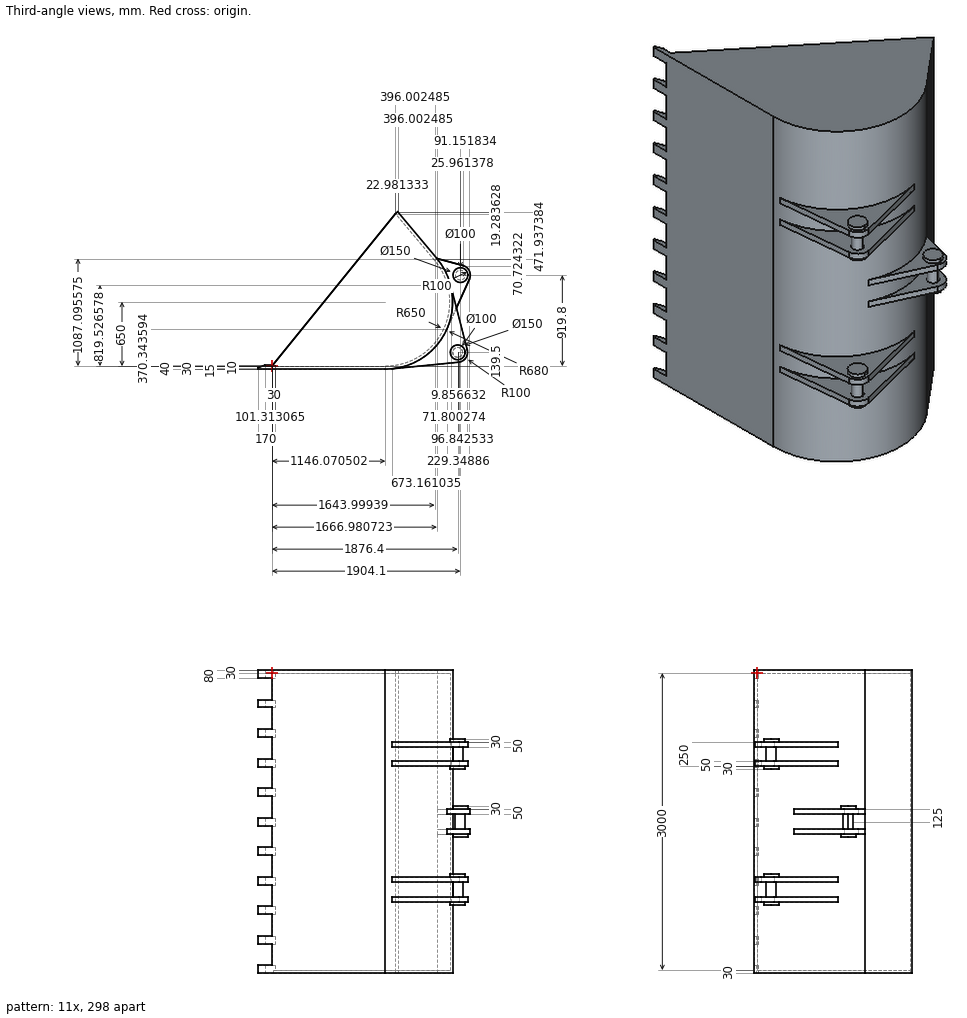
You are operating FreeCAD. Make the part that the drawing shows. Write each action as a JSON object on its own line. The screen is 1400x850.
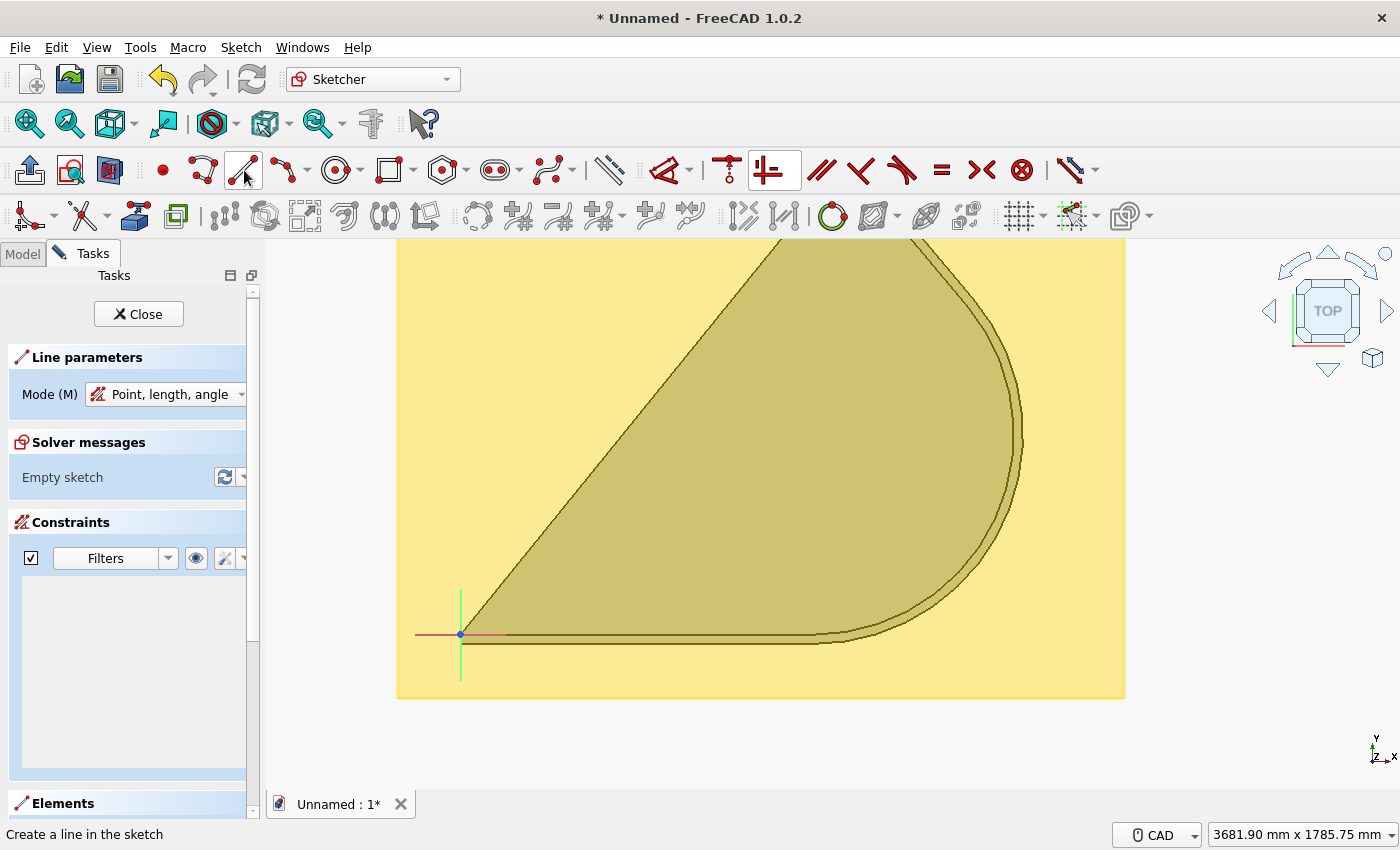
{"action": "scroll", "coordinate": [834, 643], "scroll_direction": "up", "scroll_amount": 4}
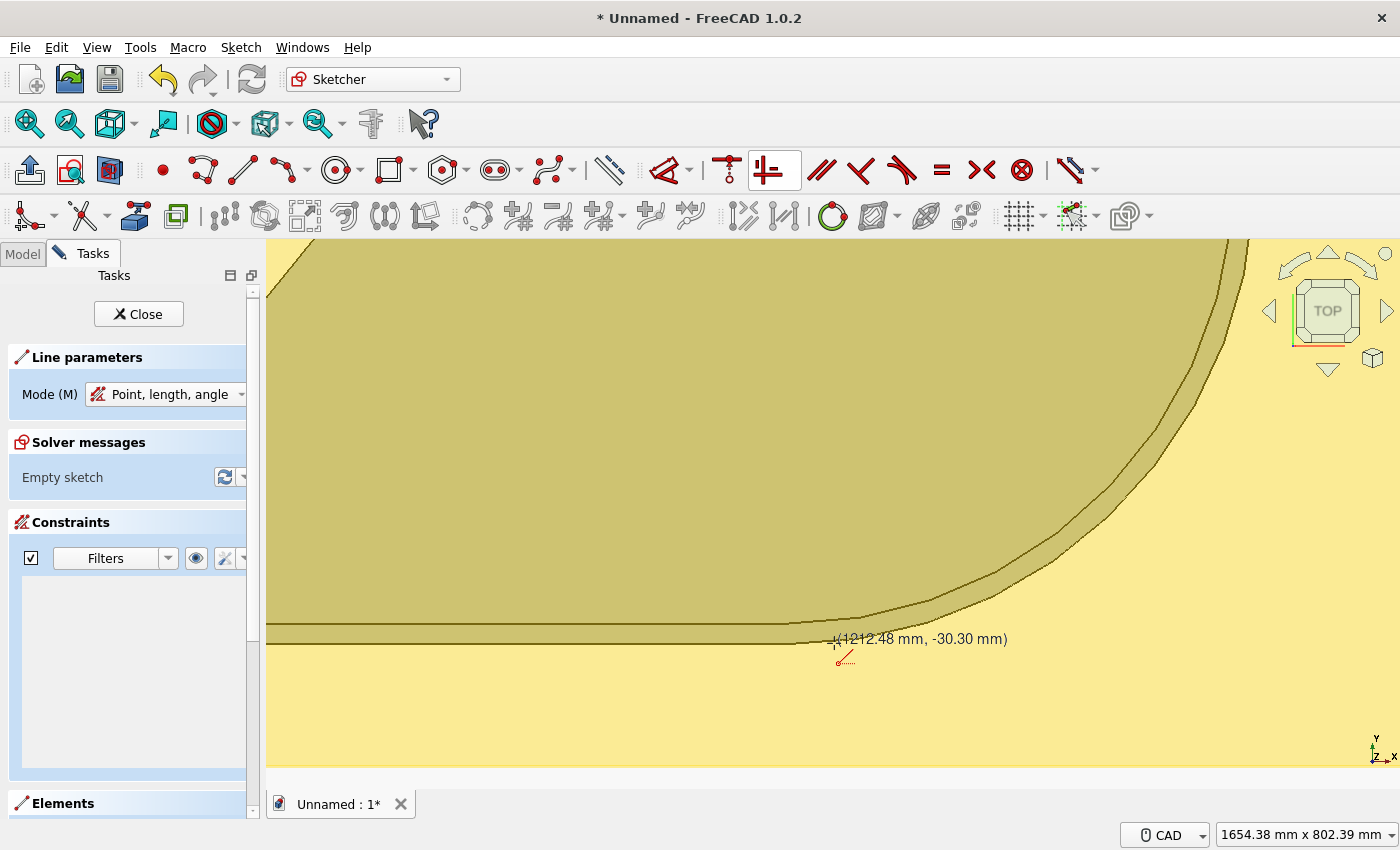
{"action": "left_click", "coordinate": [834, 642]}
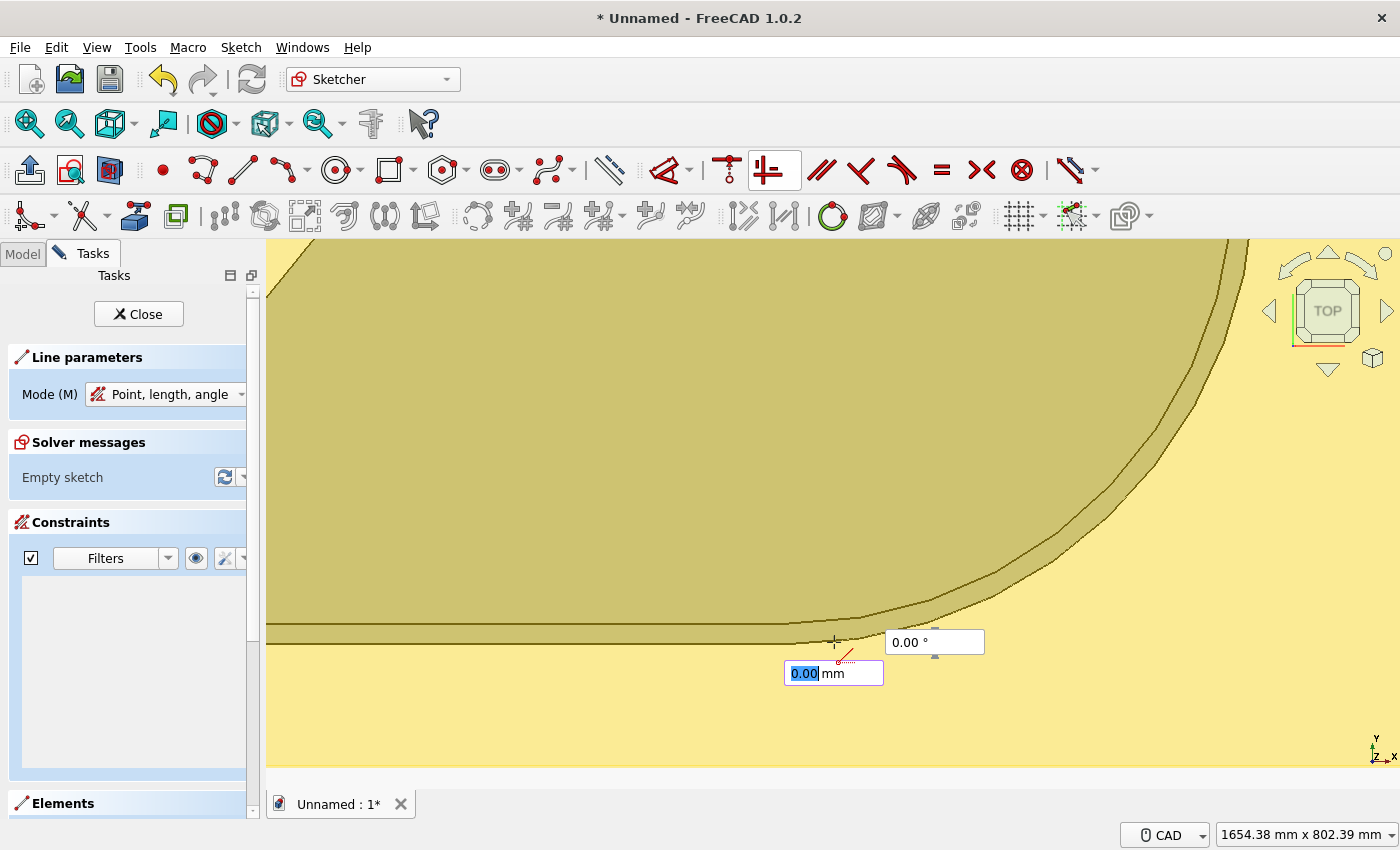
{"action": "scroll", "coordinate": [835, 646], "scroll_direction": "down", "scroll_amount": 4}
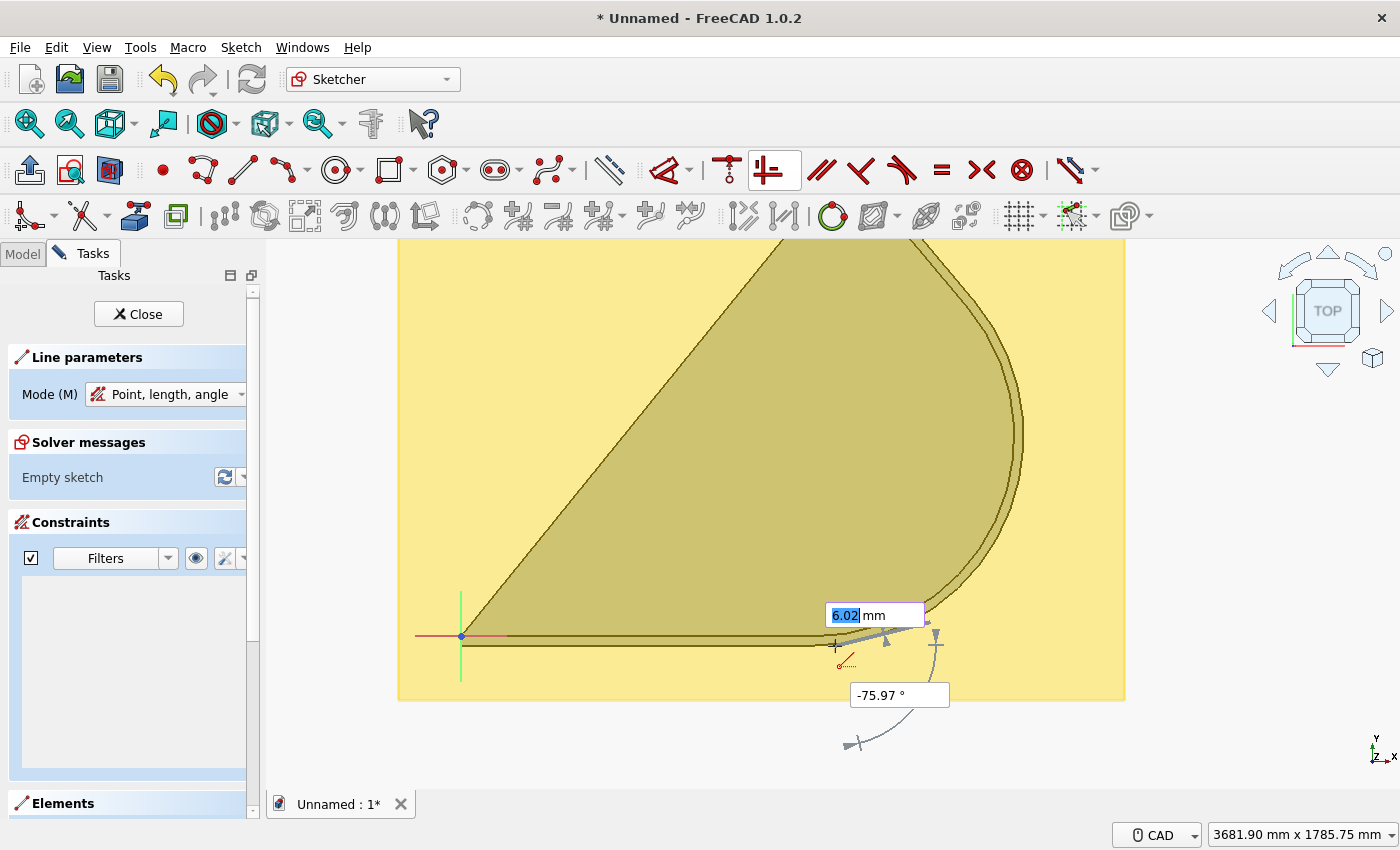
{"action": "scroll", "coordinate": [1042, 624], "scroll_direction": "up", "scroll_amount": 2}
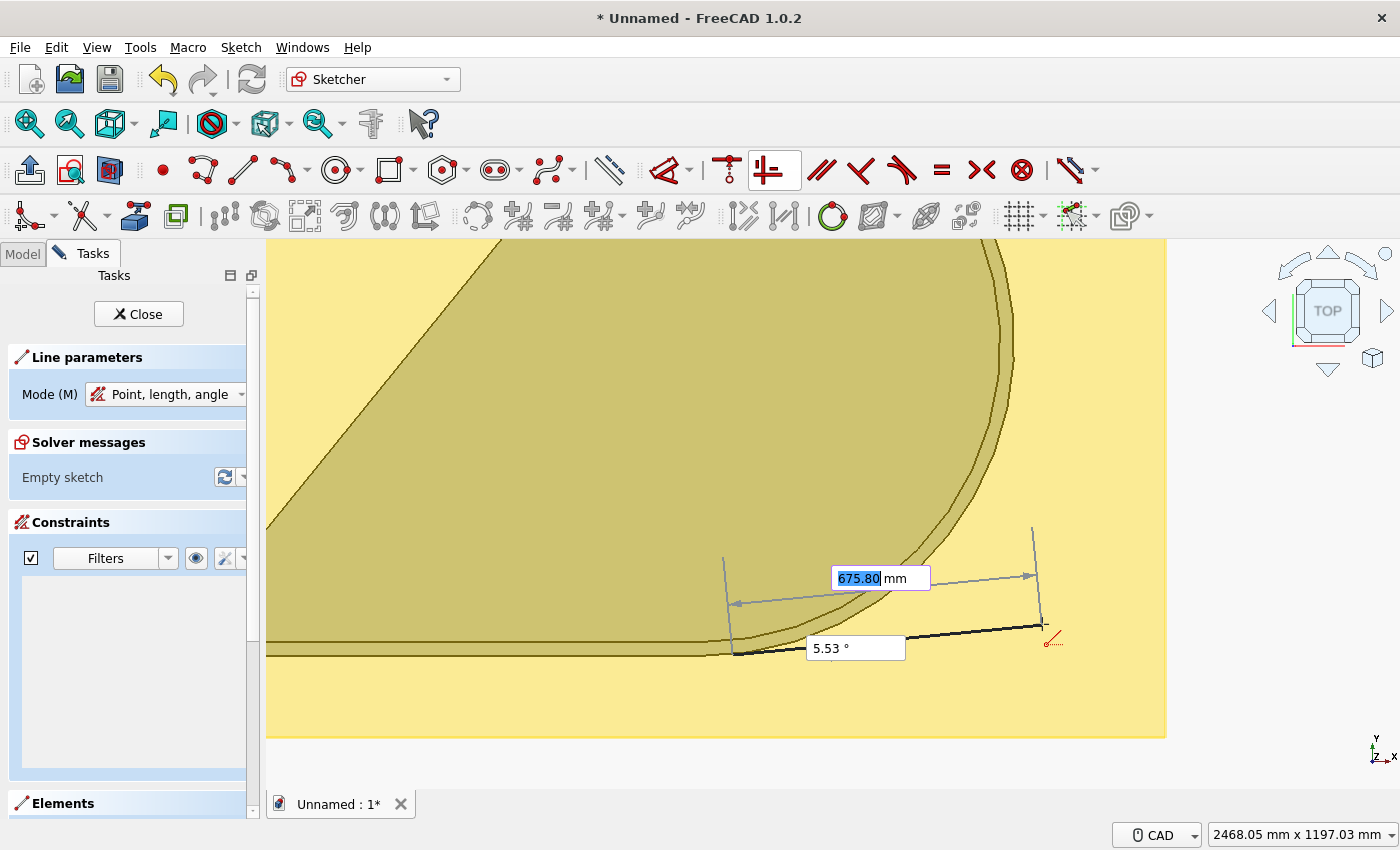
{"action": "left_click", "coordinate": [1042, 624]}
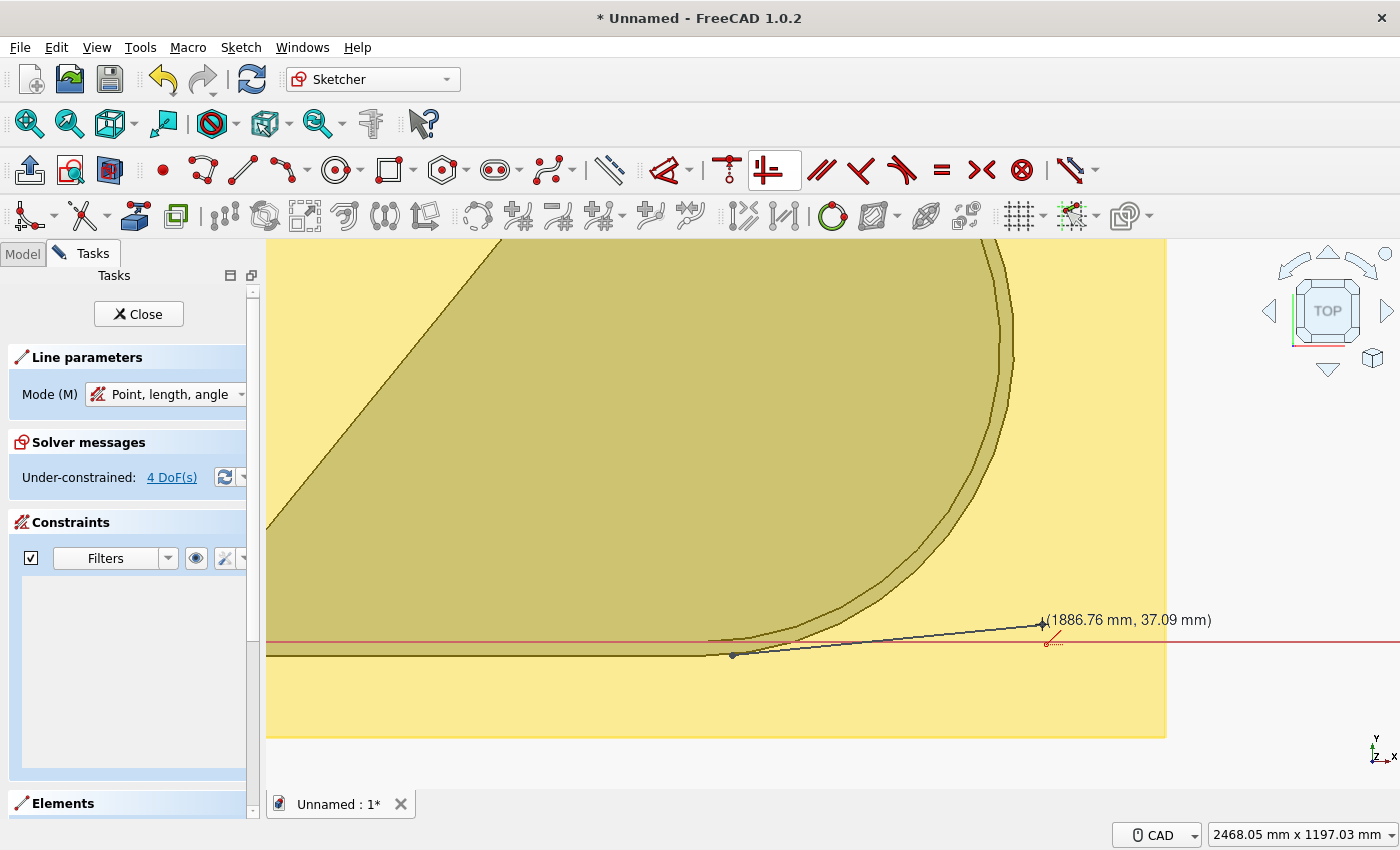
{"action": "left_click", "coordinate": [1082, 566]}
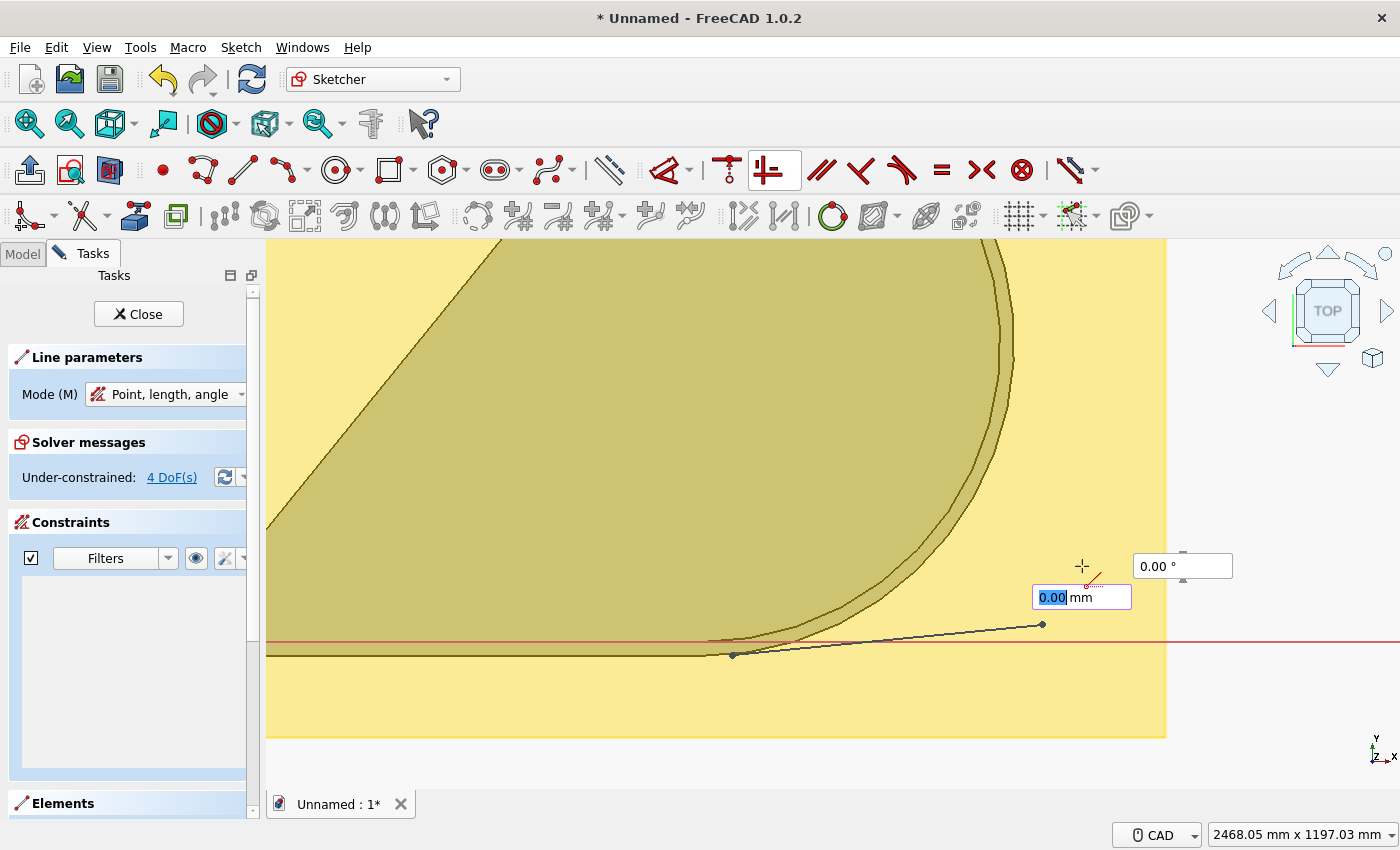
{"action": "scroll", "coordinate": [1041, 624], "scroll_direction": "down", "scroll_amount": 2}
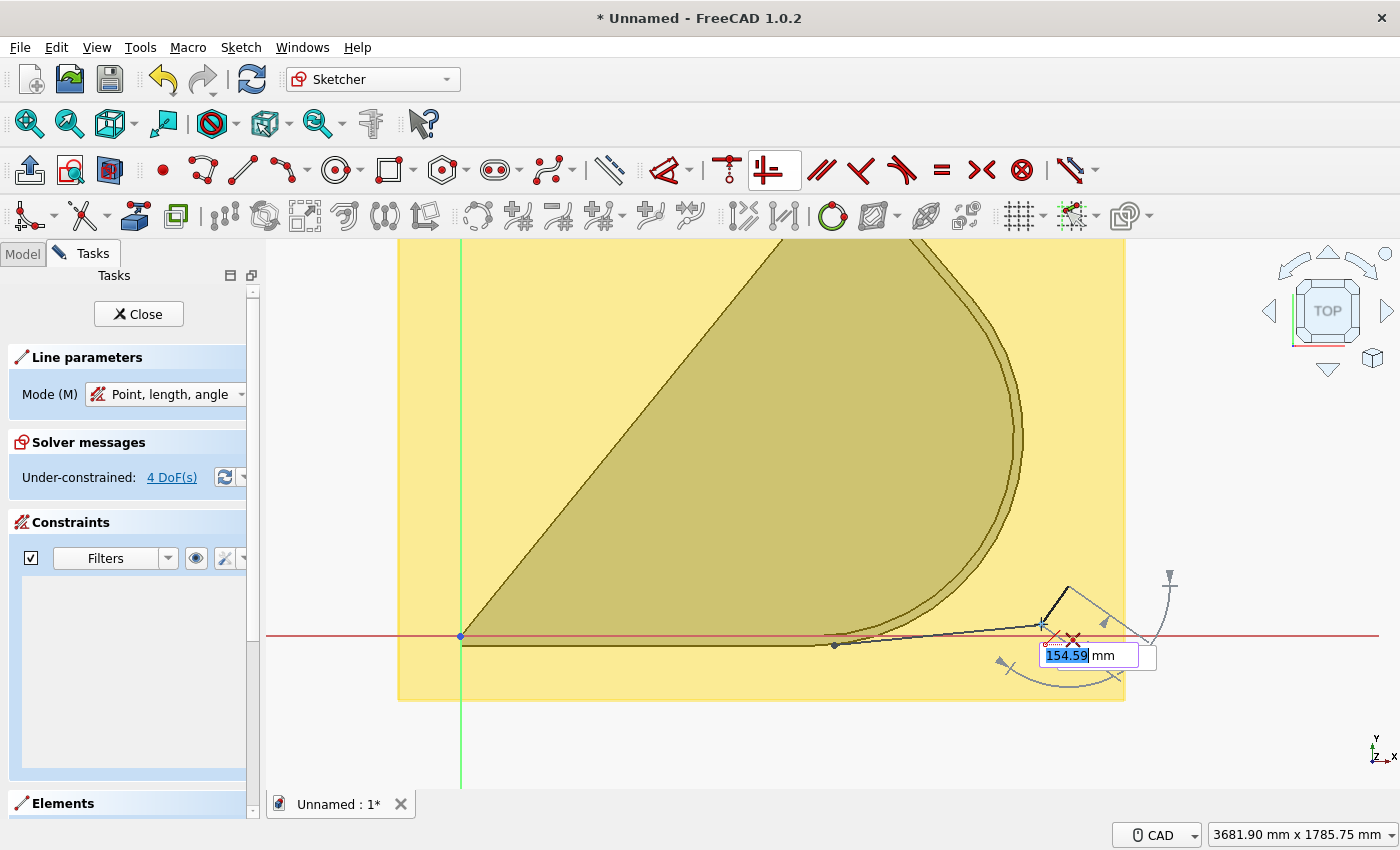
{"action": "left_click", "coordinate": [1017, 384]}